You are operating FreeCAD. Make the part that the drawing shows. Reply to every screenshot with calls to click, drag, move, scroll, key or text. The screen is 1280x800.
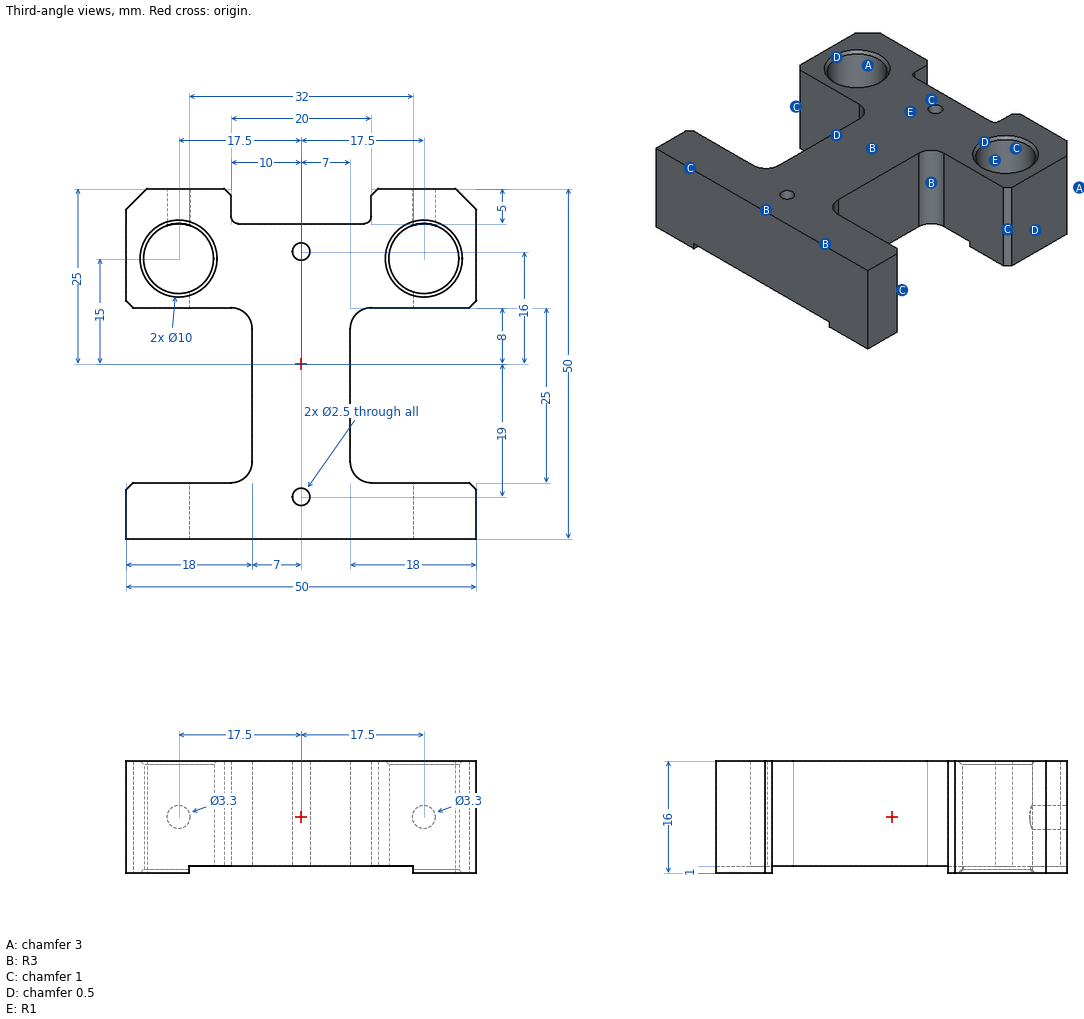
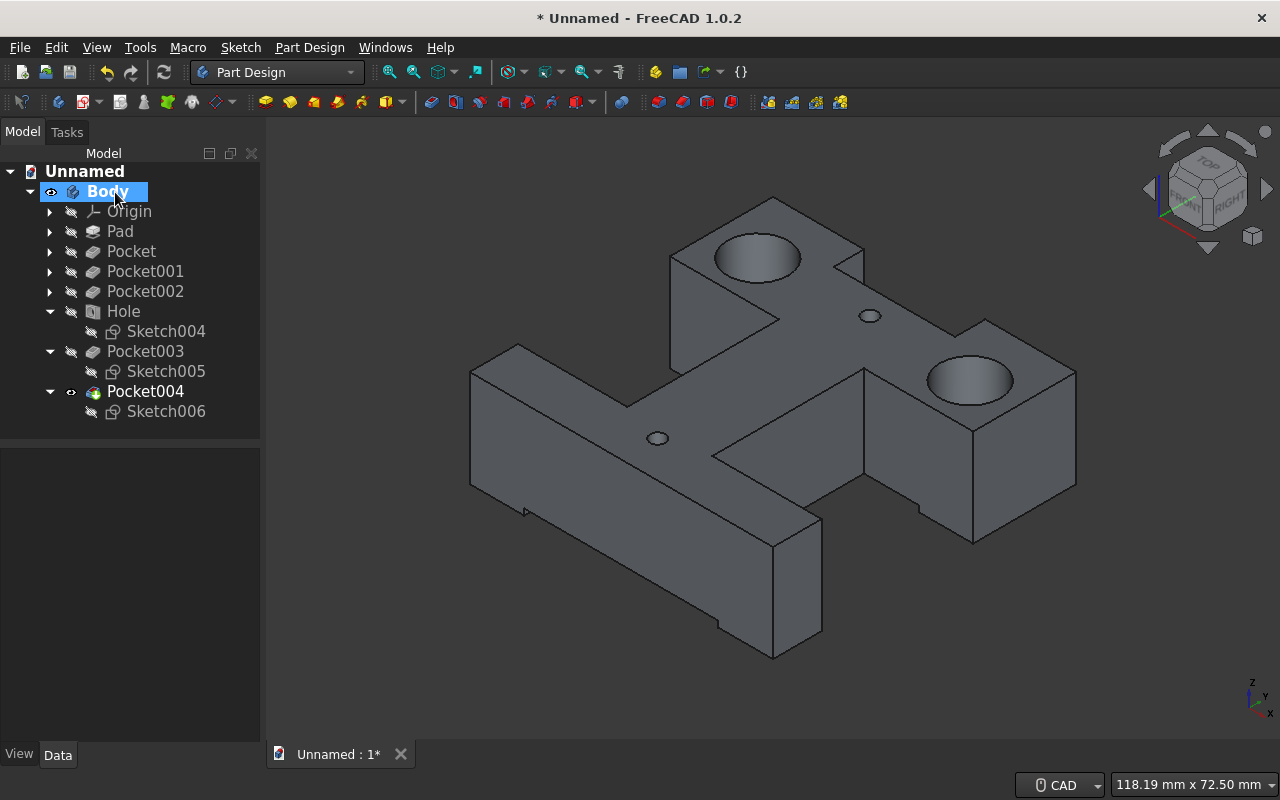
key(2)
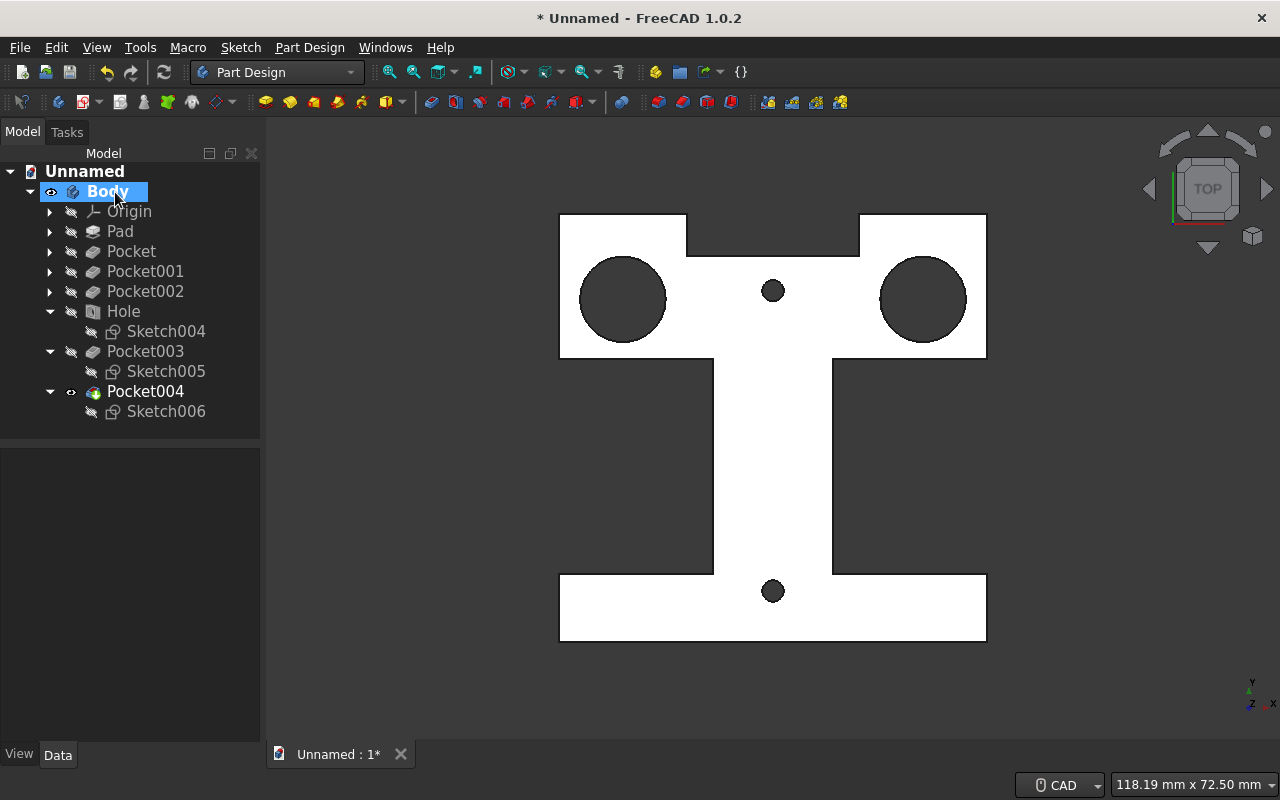
key(0)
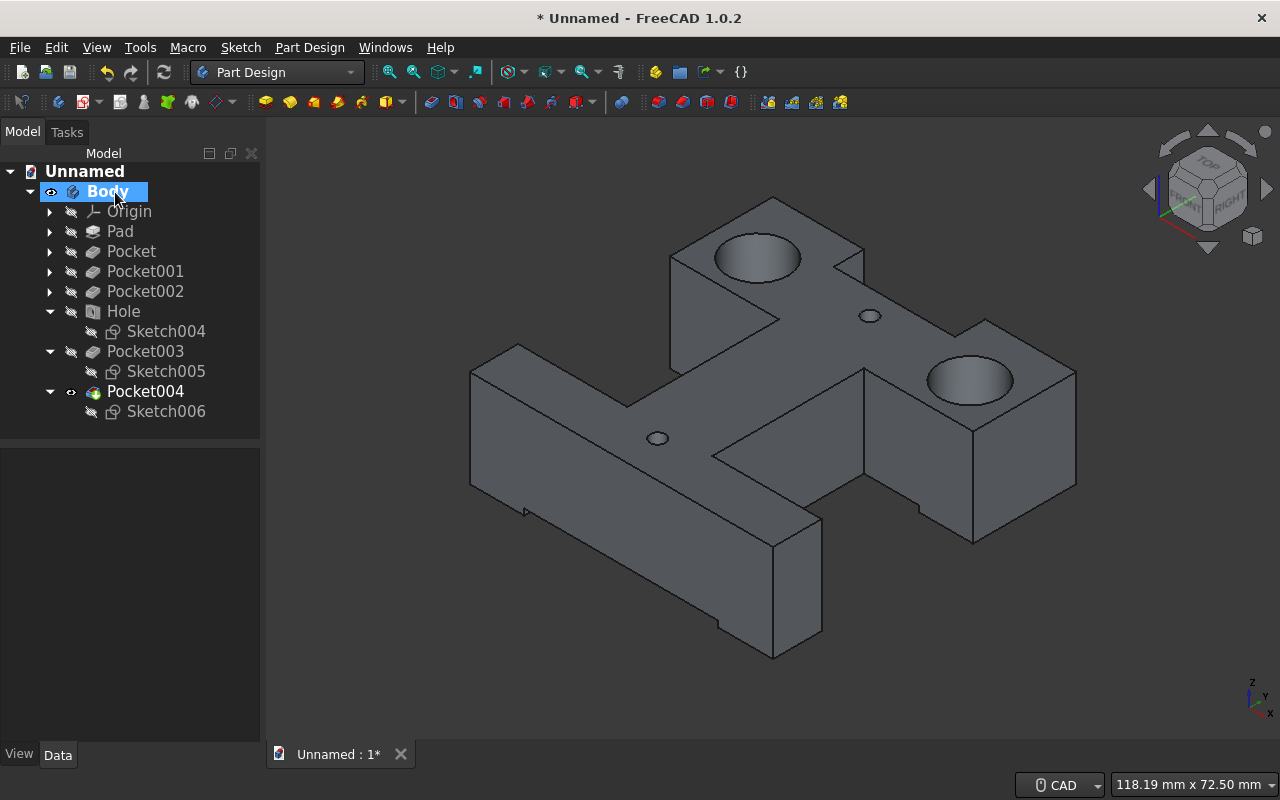
key(1)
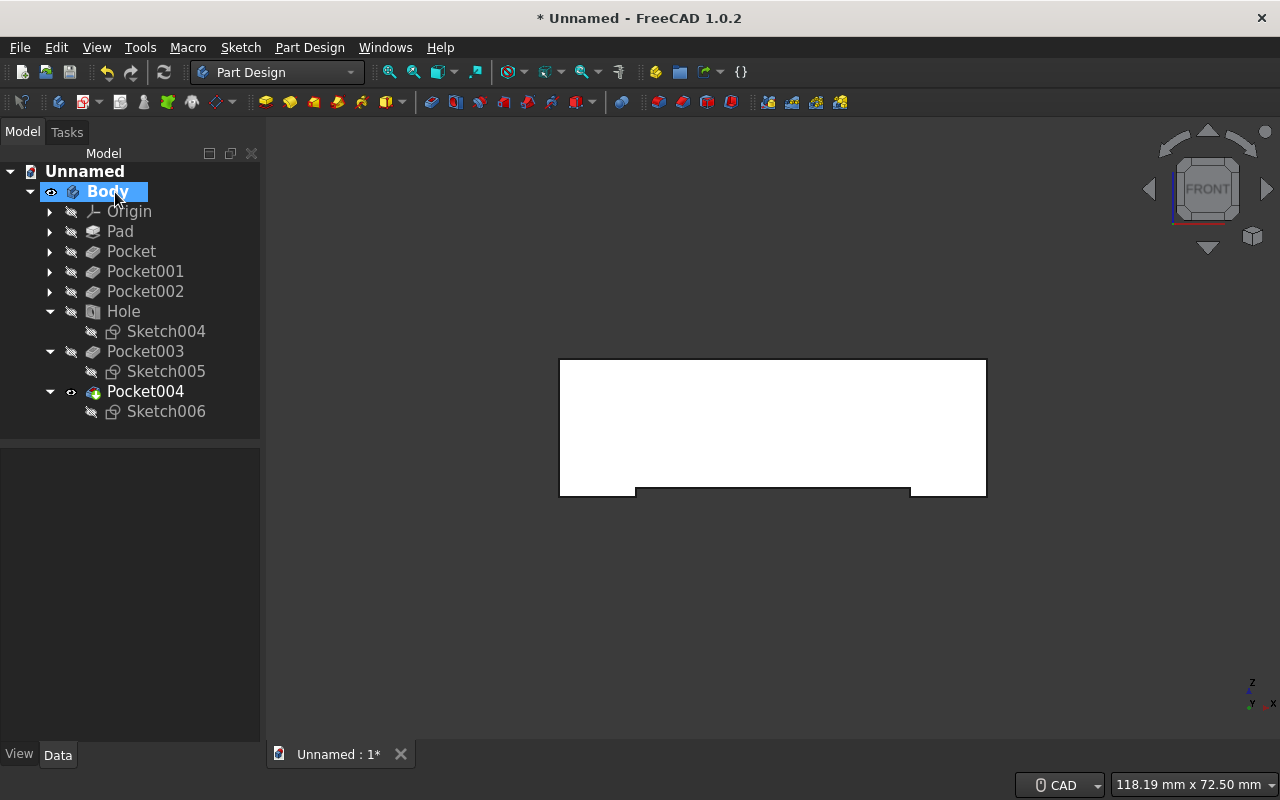
key(v)
key(f)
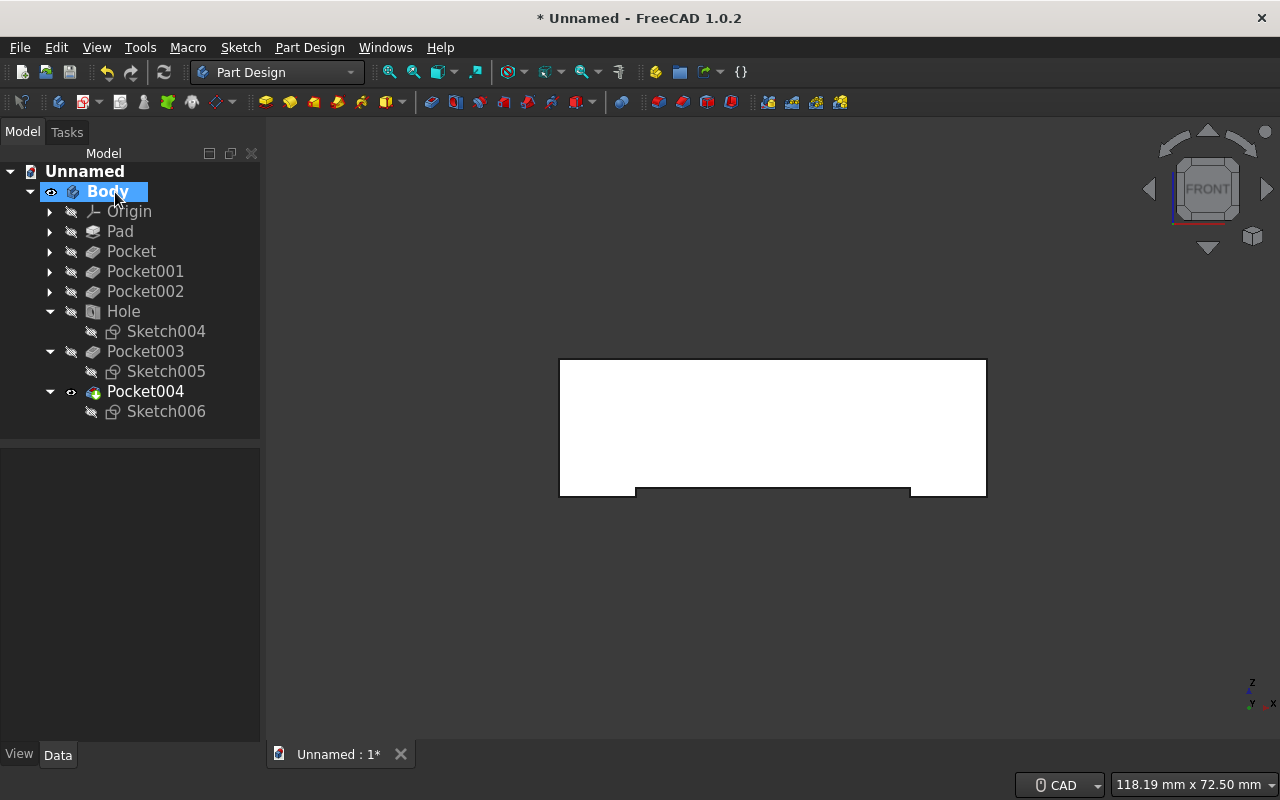
key(3)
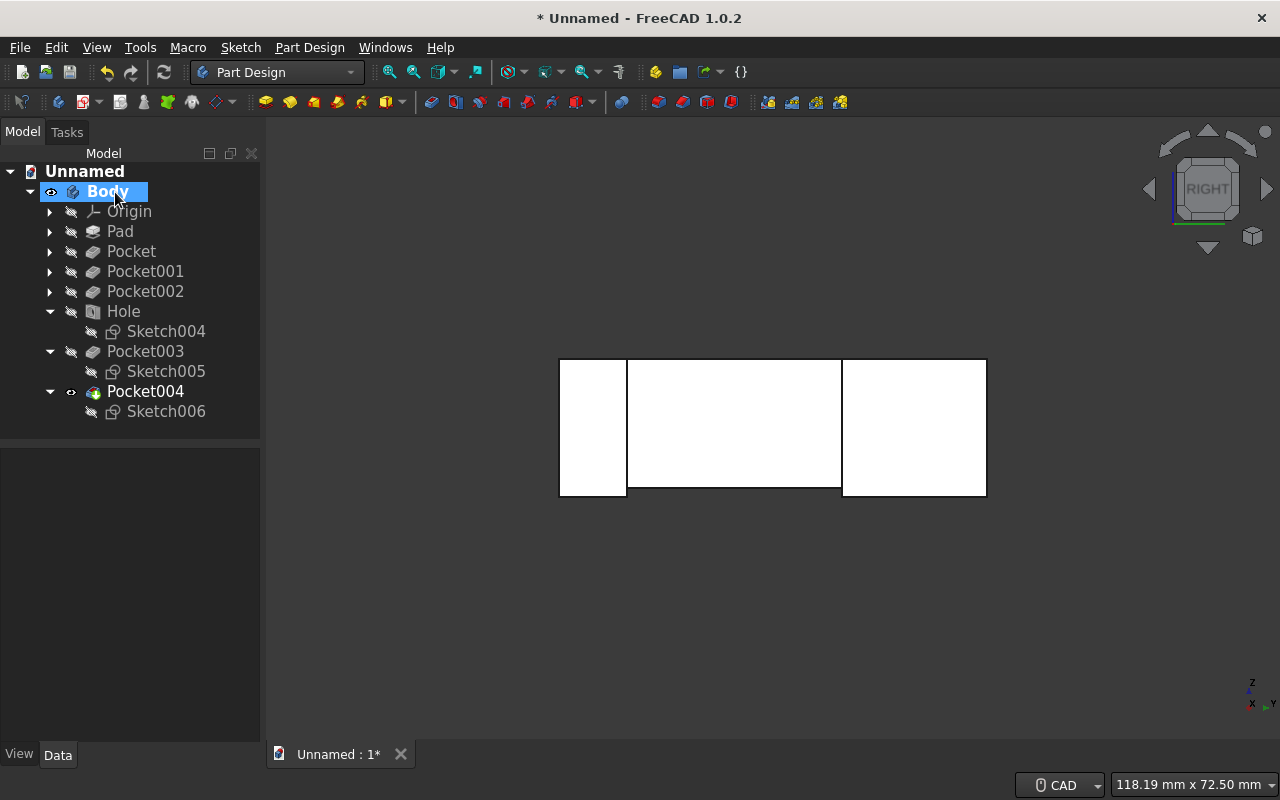
key(v)
key(f)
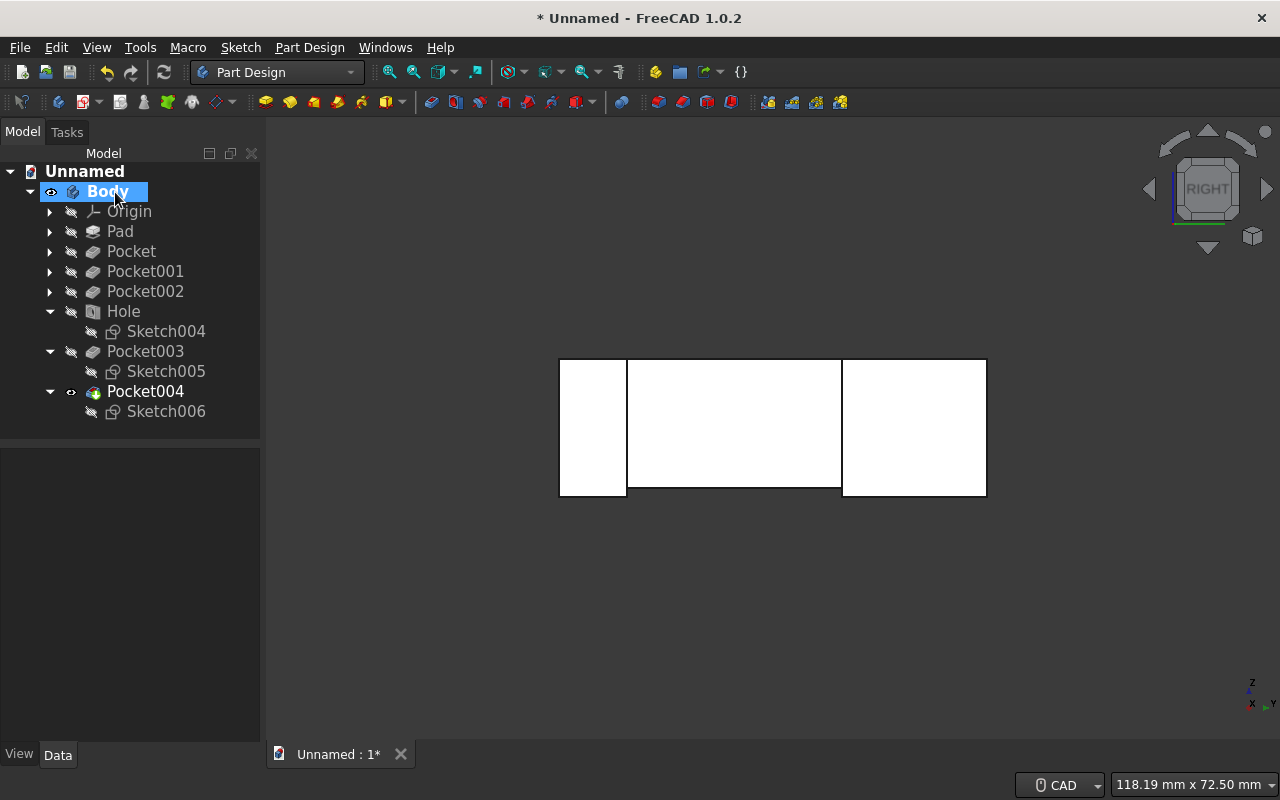
click(987, 427)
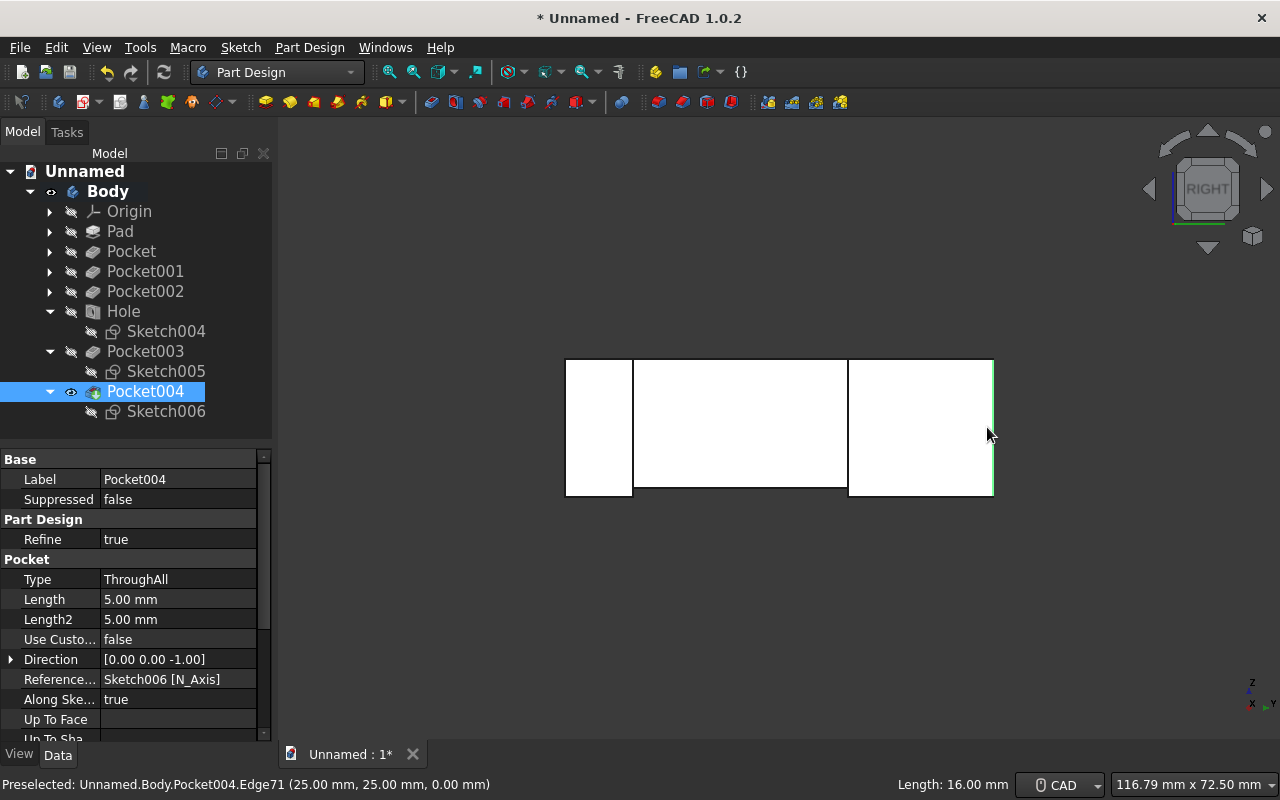
key(5)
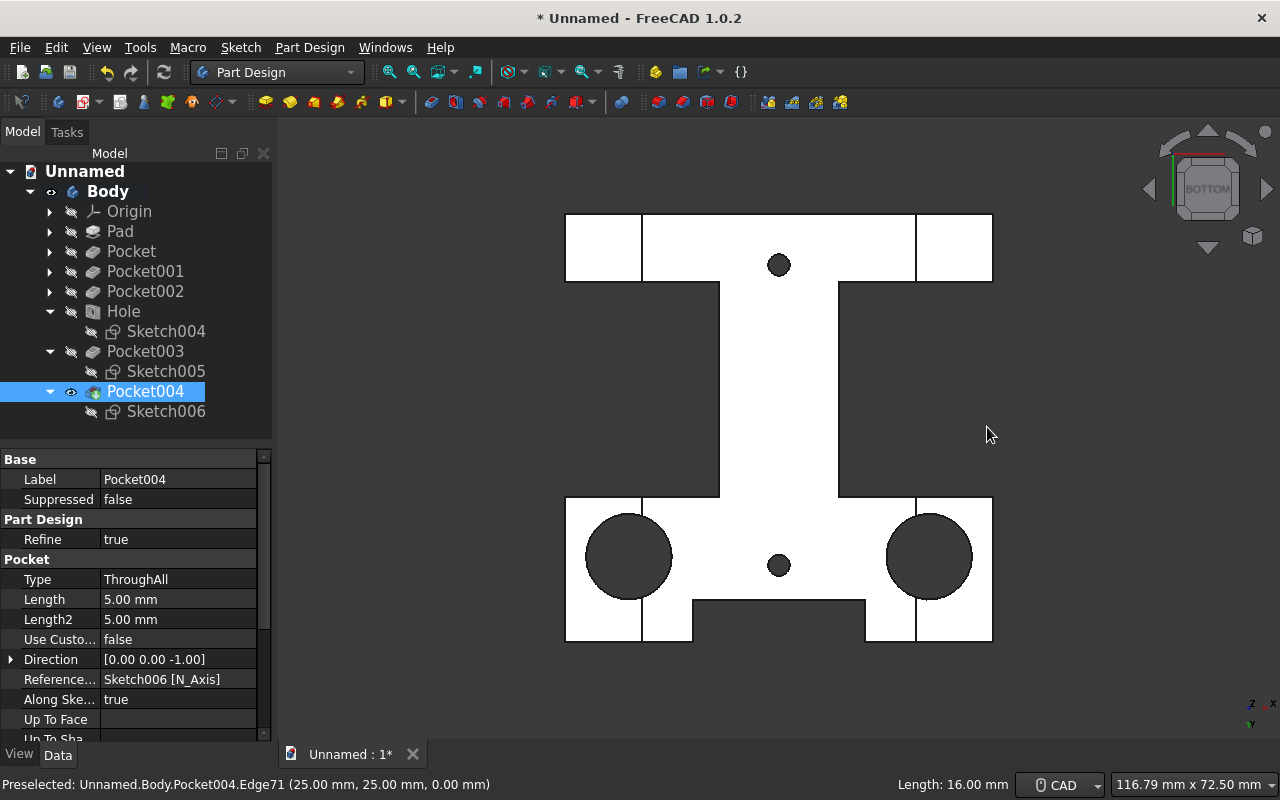
key(4)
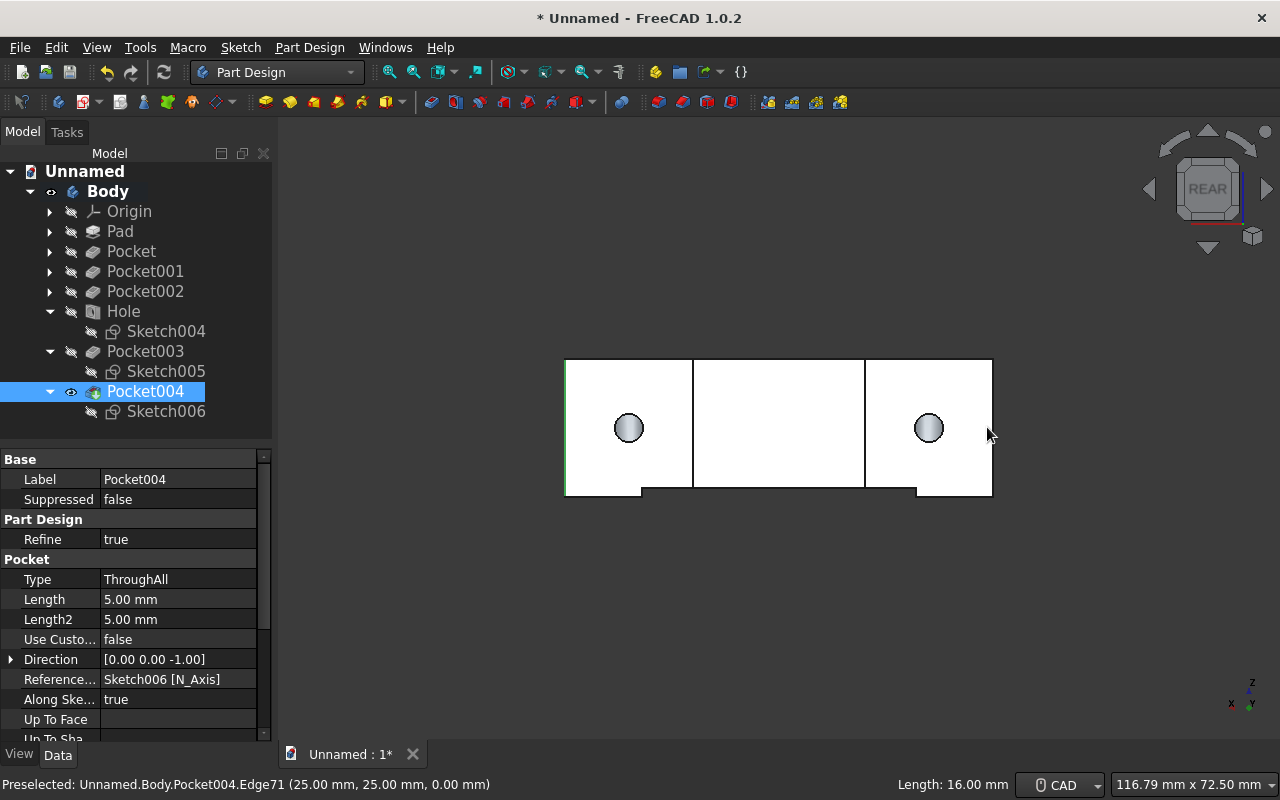
click(390, 72)